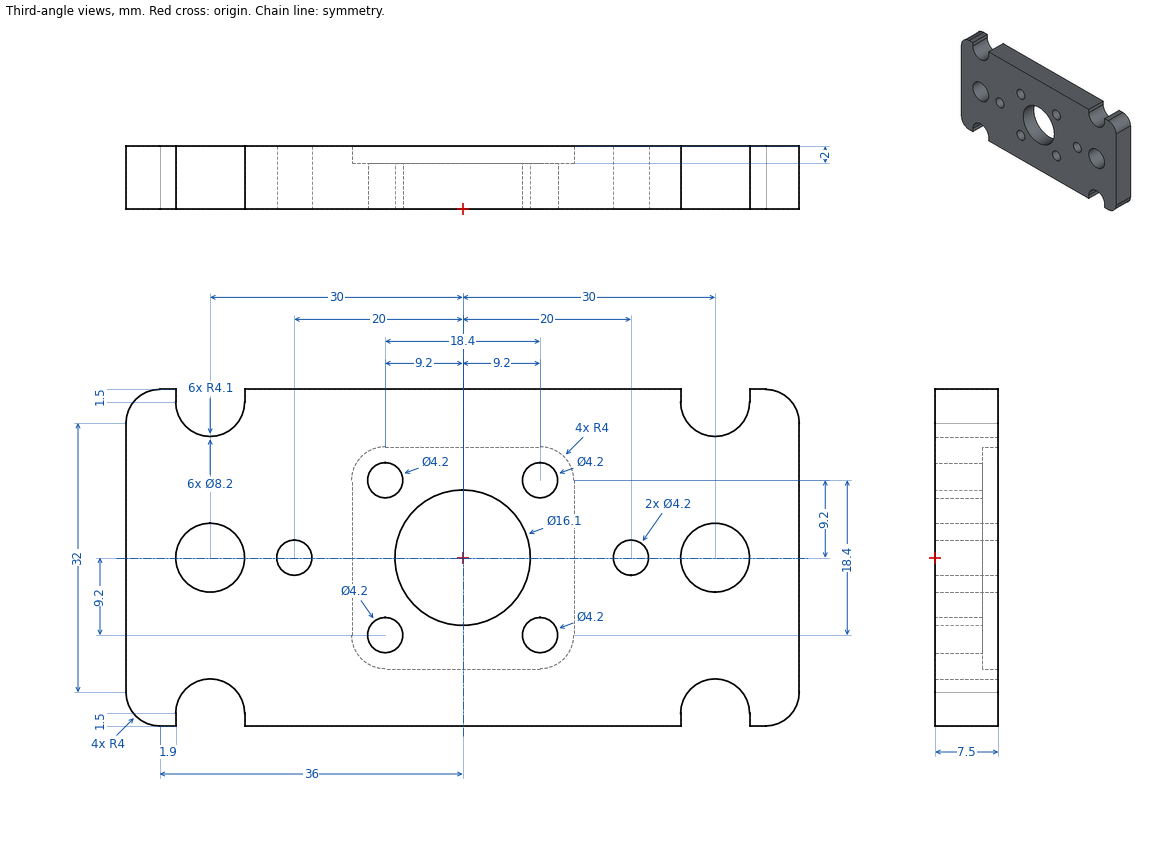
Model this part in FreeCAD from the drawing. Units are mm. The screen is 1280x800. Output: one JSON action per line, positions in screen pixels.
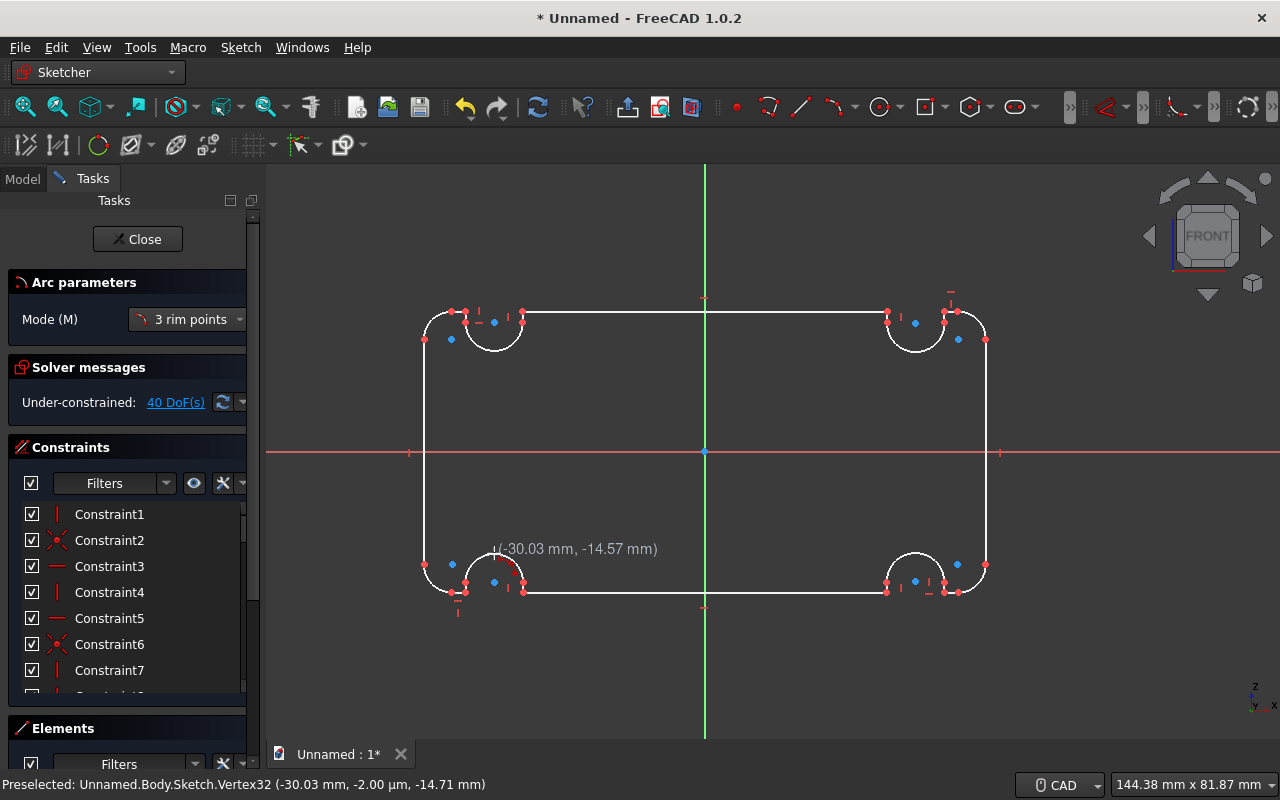
{"action": "left_click", "coordinate": [880, 108]}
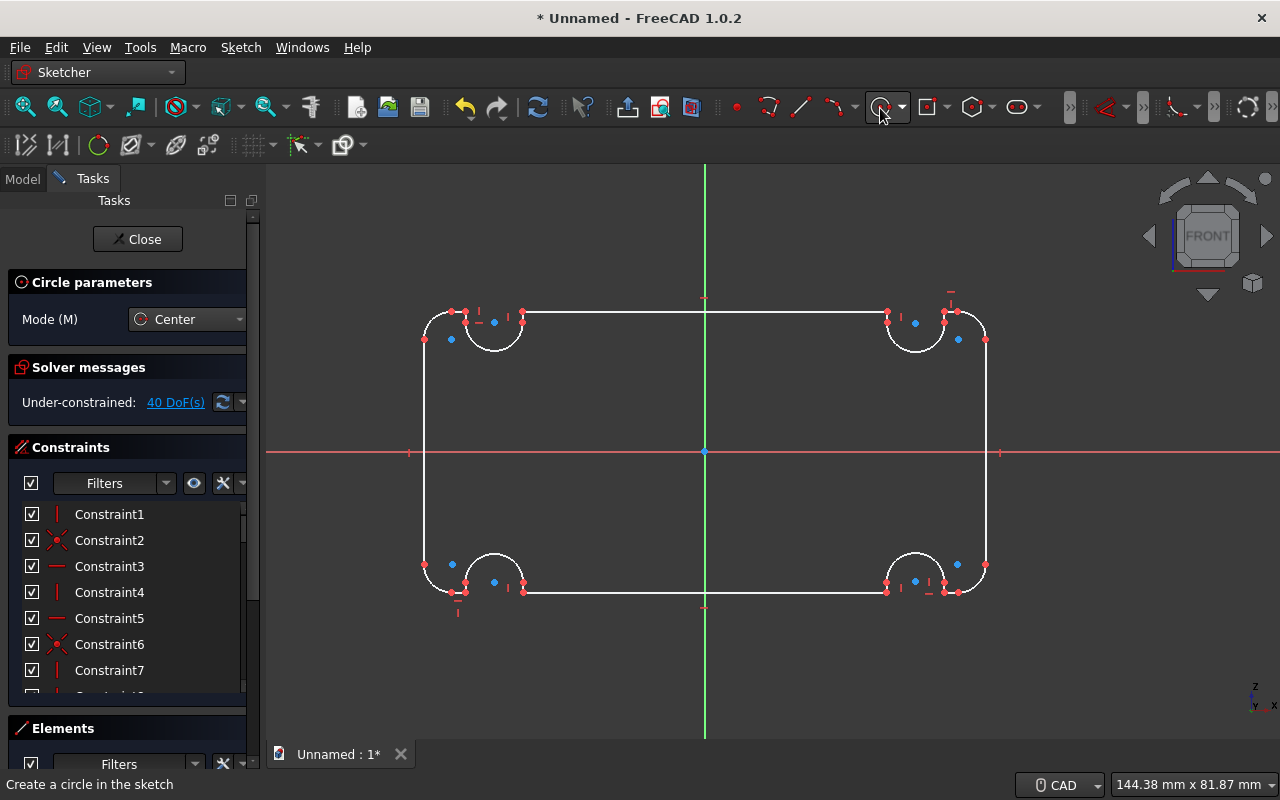
{"action": "left_click", "coordinate": [916, 452]}
{"action": "mouse_move", "coordinate": [936, 431]}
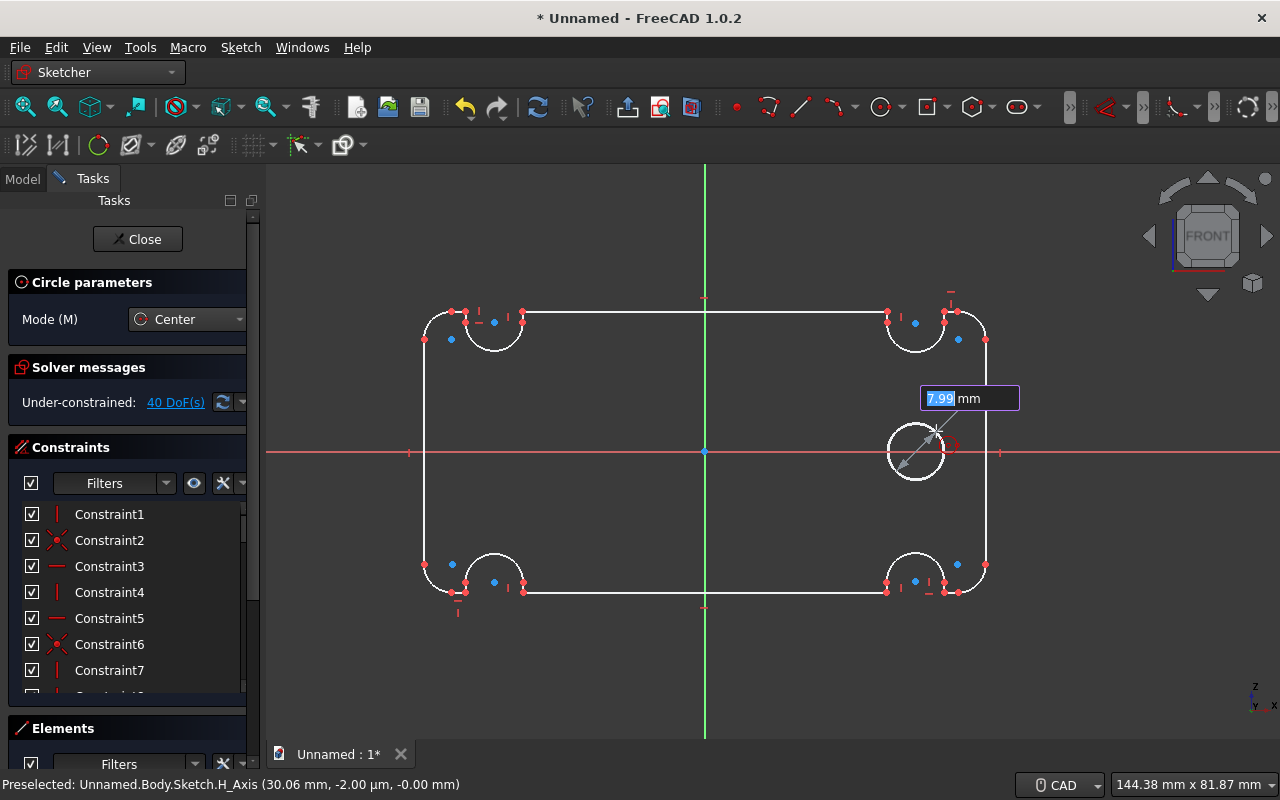
{"action": "type", "text": "8.2"}
{"action": "key", "text": "Return"}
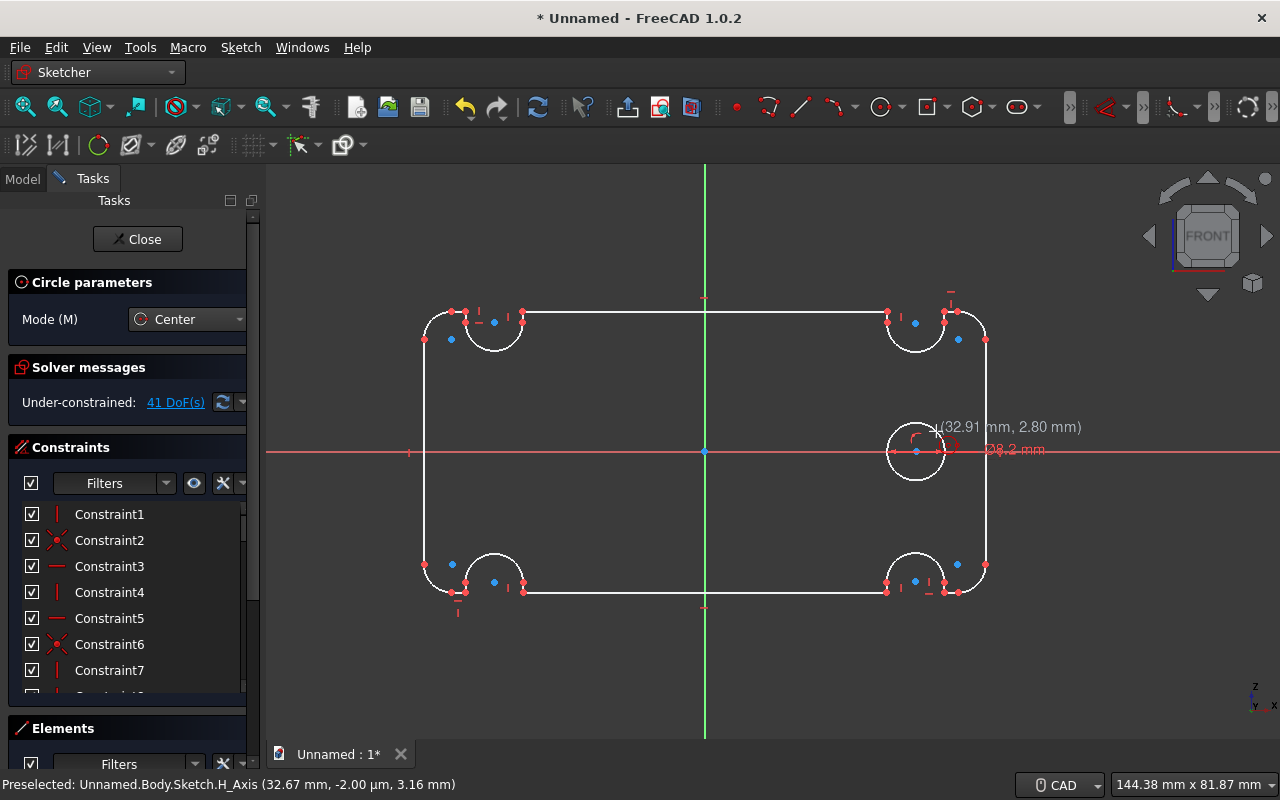
{"action": "scroll", "coordinate": [845, 452], "scroll_direction": "up", "scroll_amount": 3}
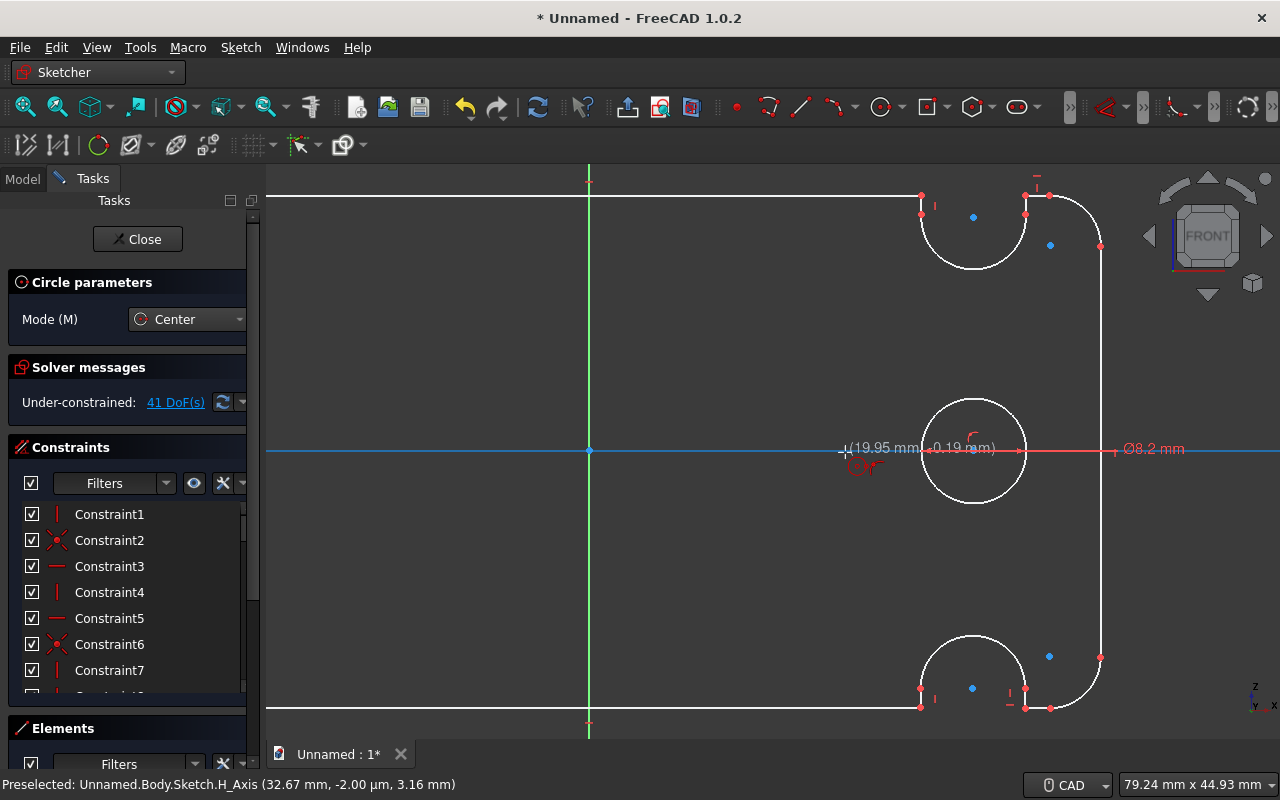
{"action": "left_click", "coordinate": [845, 451]}
{"action": "mouse_move", "coordinate": [864, 432]}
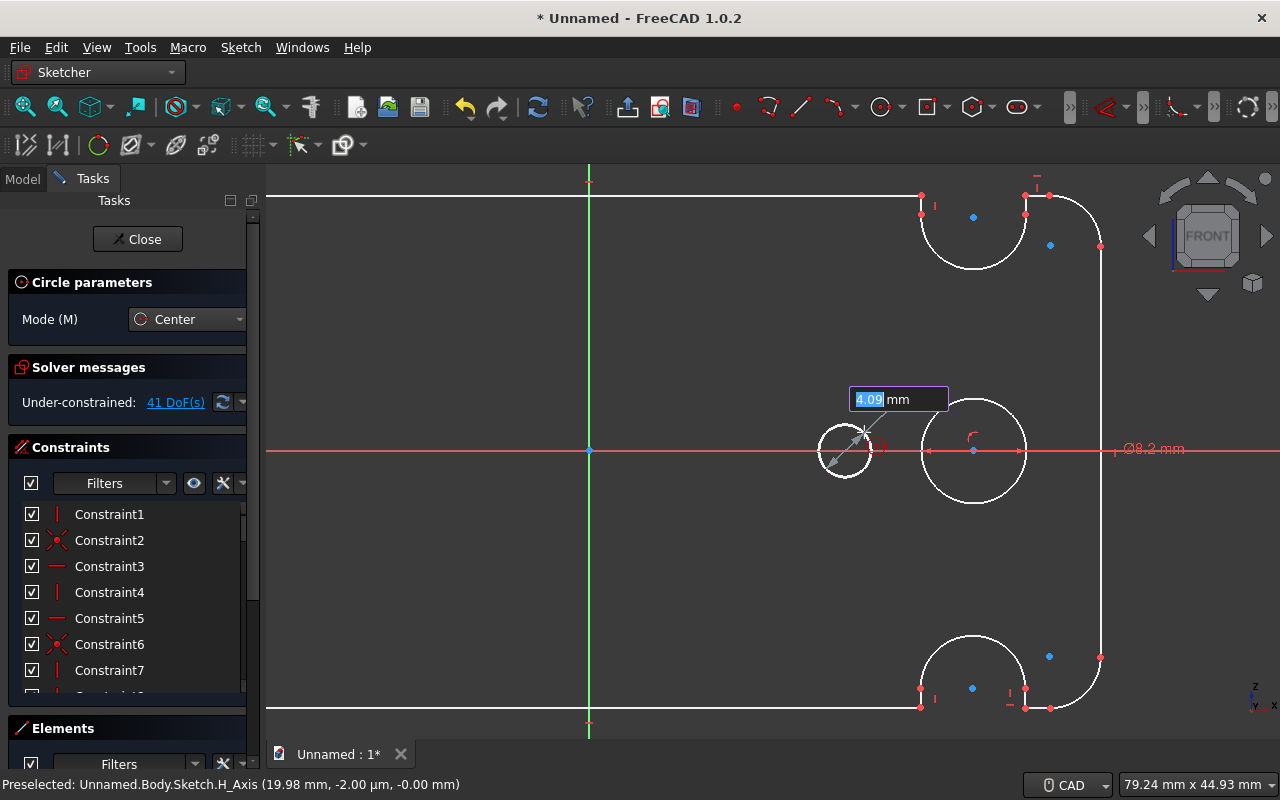
{"action": "type", "text": "4.2"}
{"action": "key", "text": "Return"}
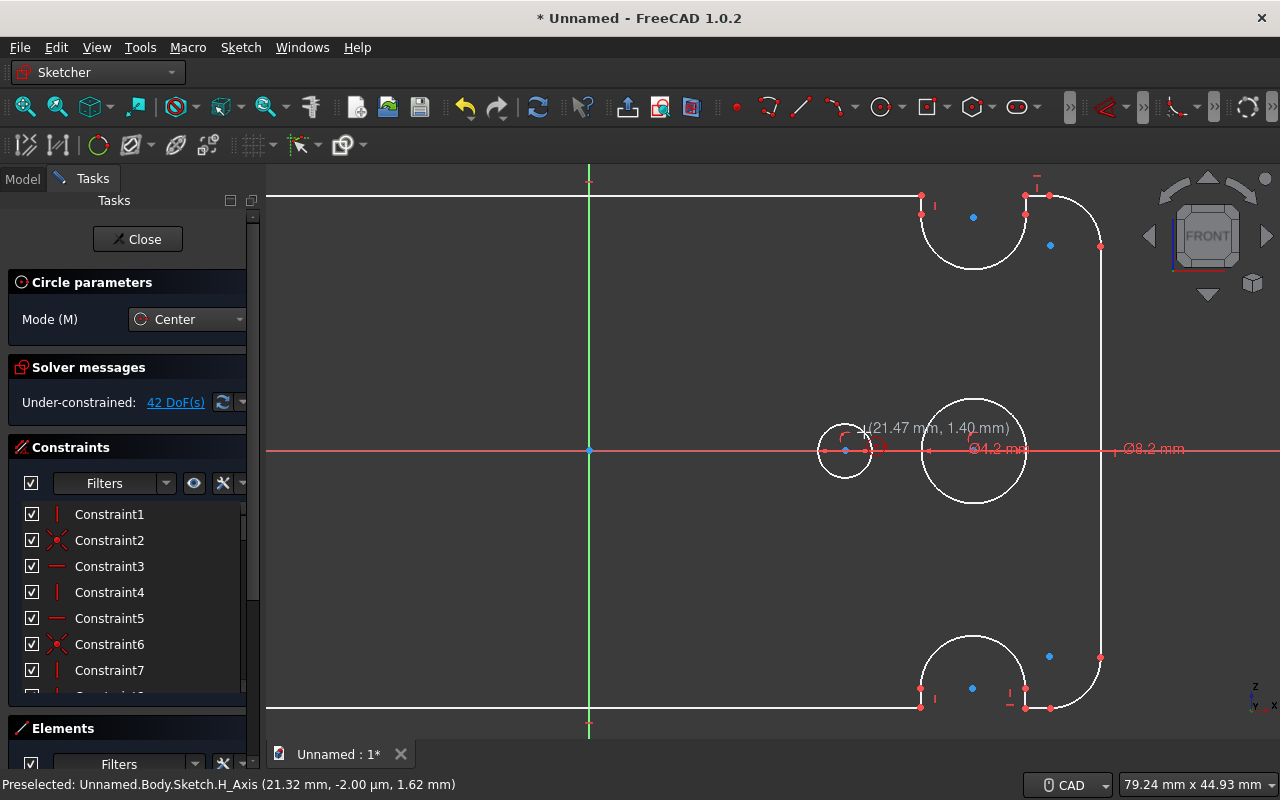
{"action": "left_click", "coordinate": [333, 451]}
{"action": "mouse_move", "coordinate": [352, 432]}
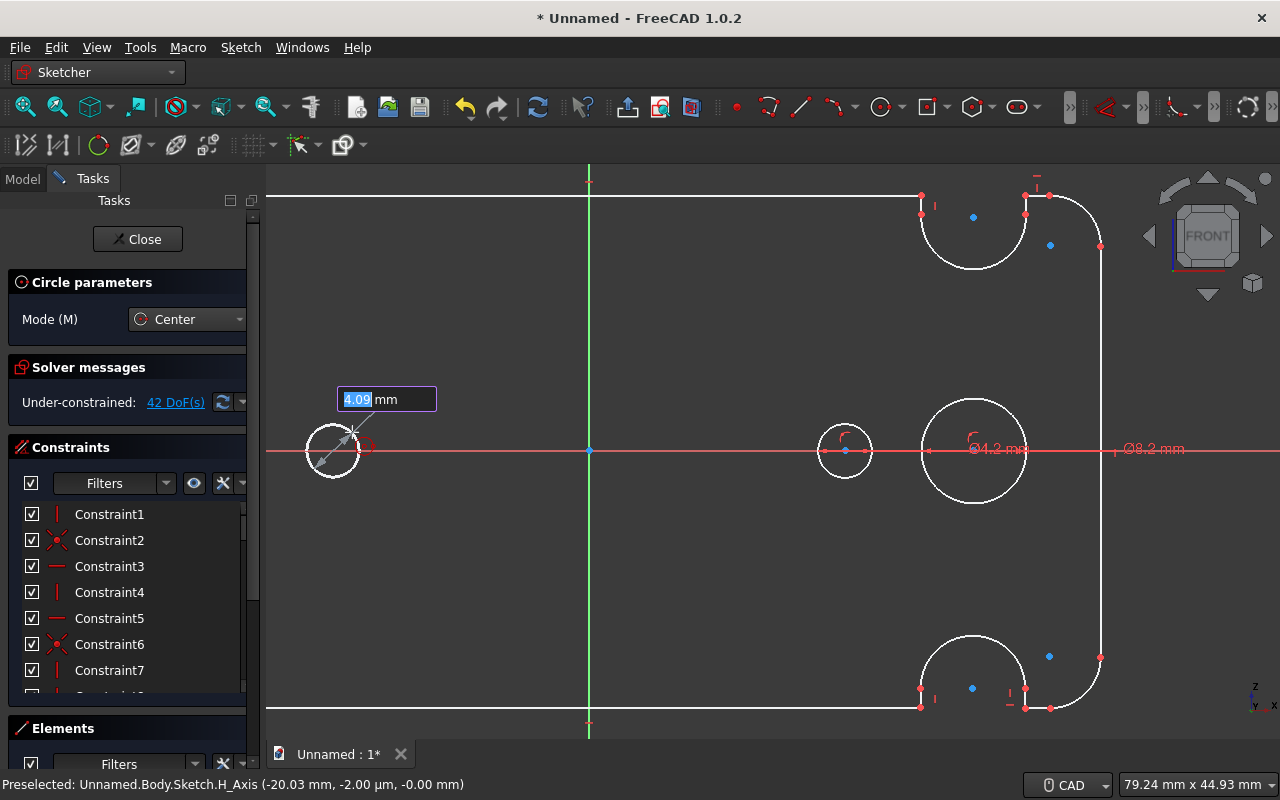
{"action": "type", "text": "4.2"}
{"action": "key", "text": "Return"}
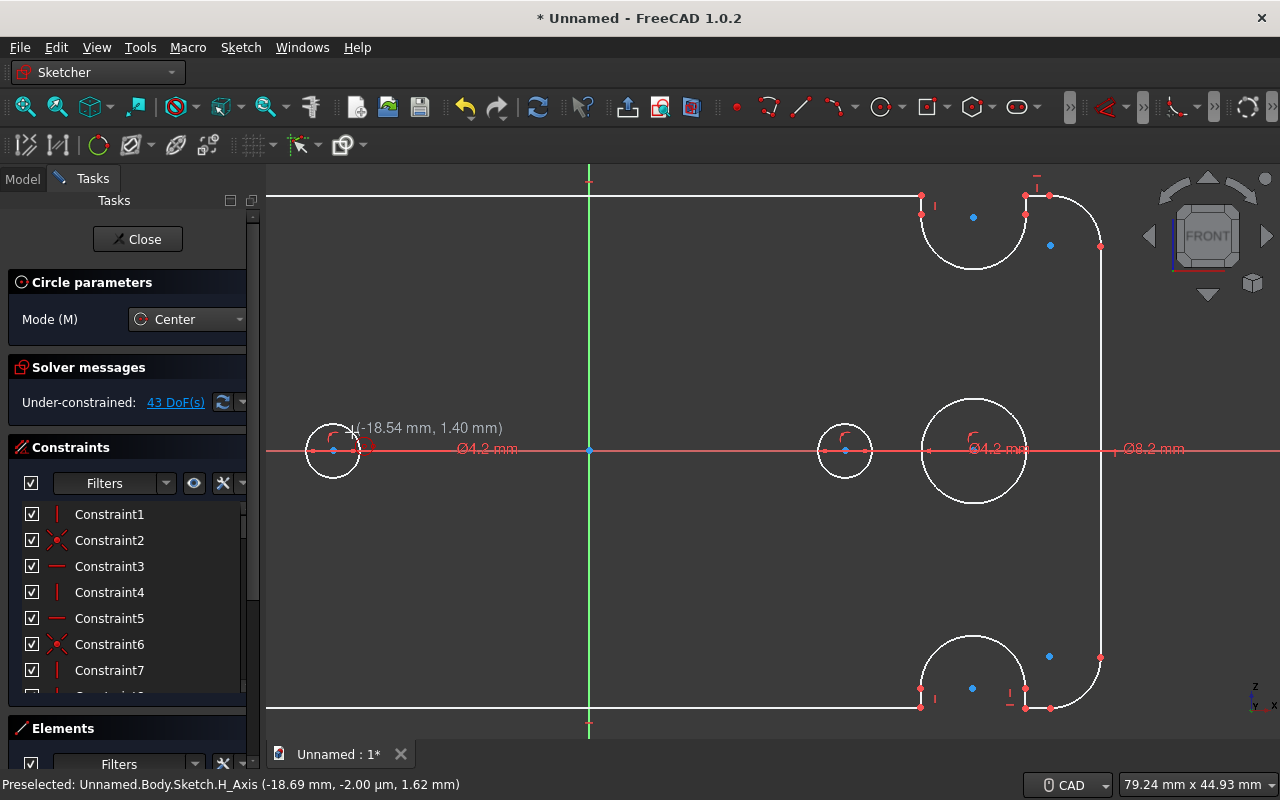
{"action": "scroll", "coordinate": [845, 452], "scroll_direction": "down", "scroll_amount": 3}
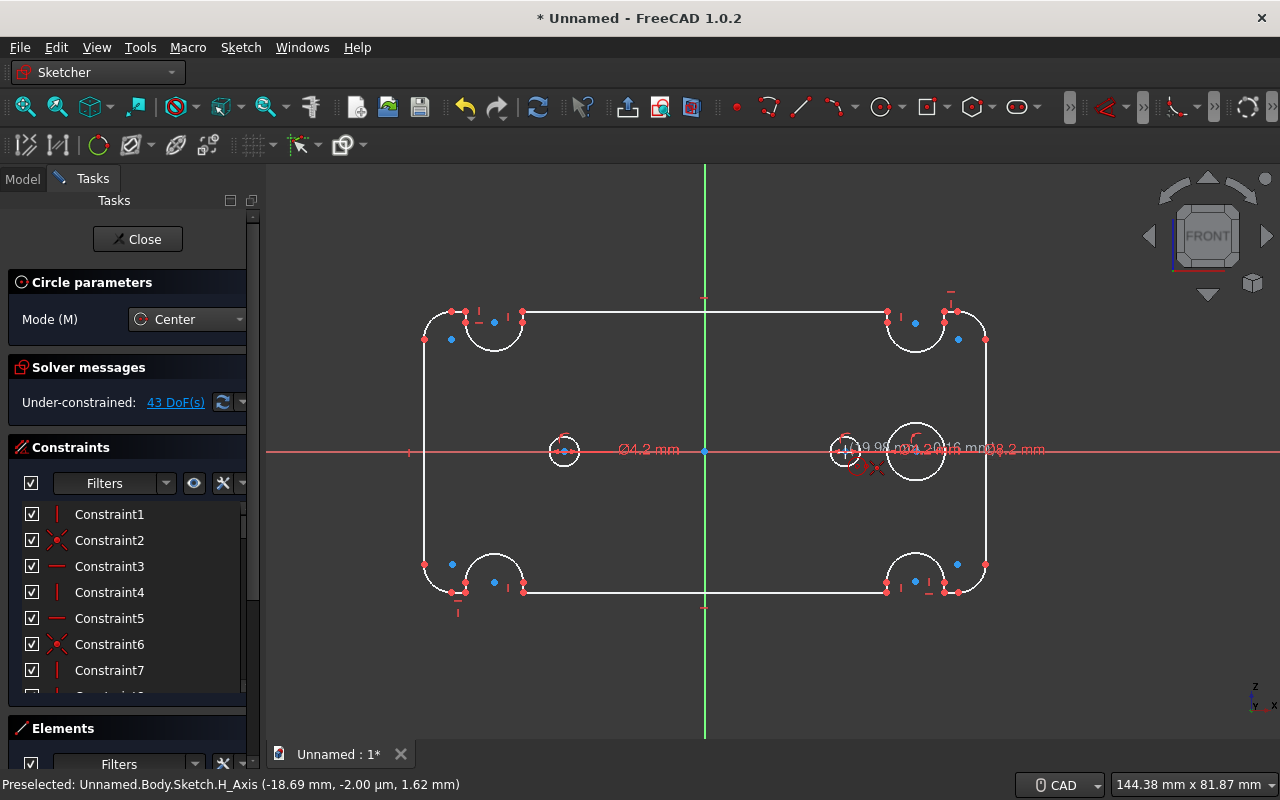
{"action": "left_click", "coordinate": [494, 452]}
{"action": "mouse_move", "coordinate": [515, 431]}